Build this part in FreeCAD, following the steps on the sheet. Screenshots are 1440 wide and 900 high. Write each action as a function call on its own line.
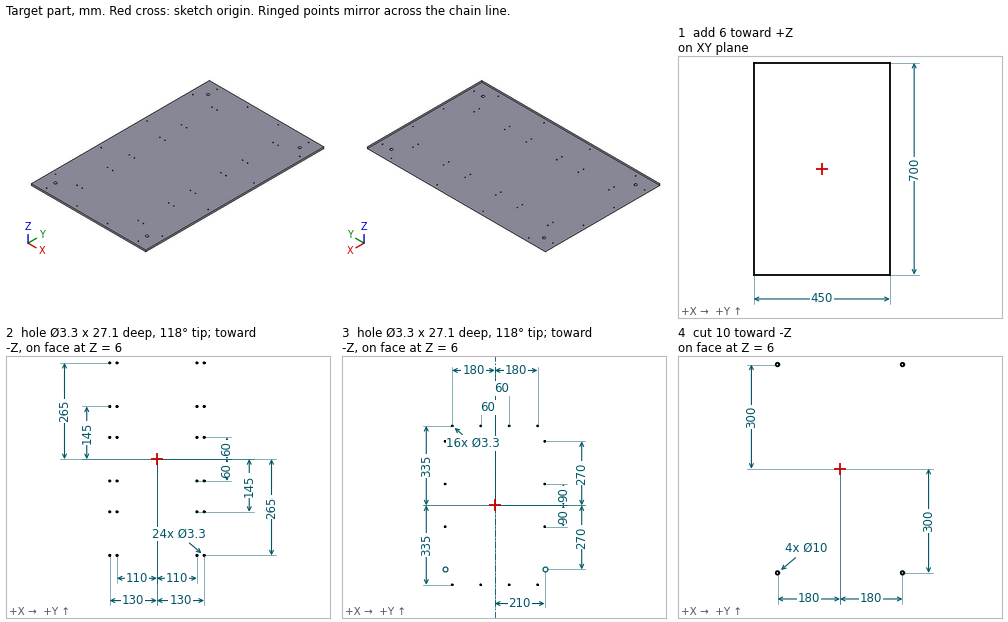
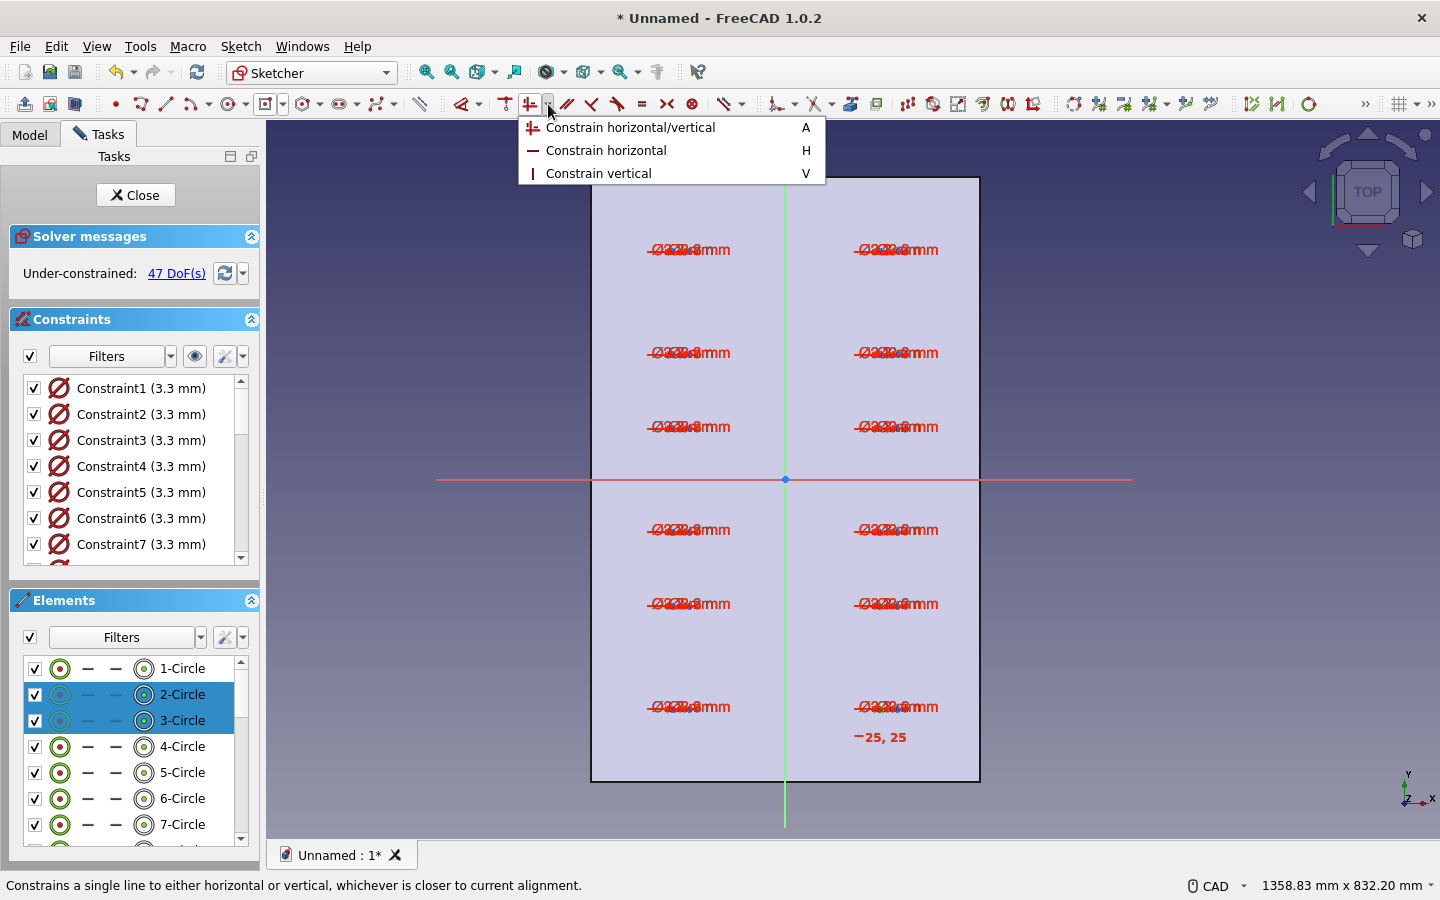
click(672, 174)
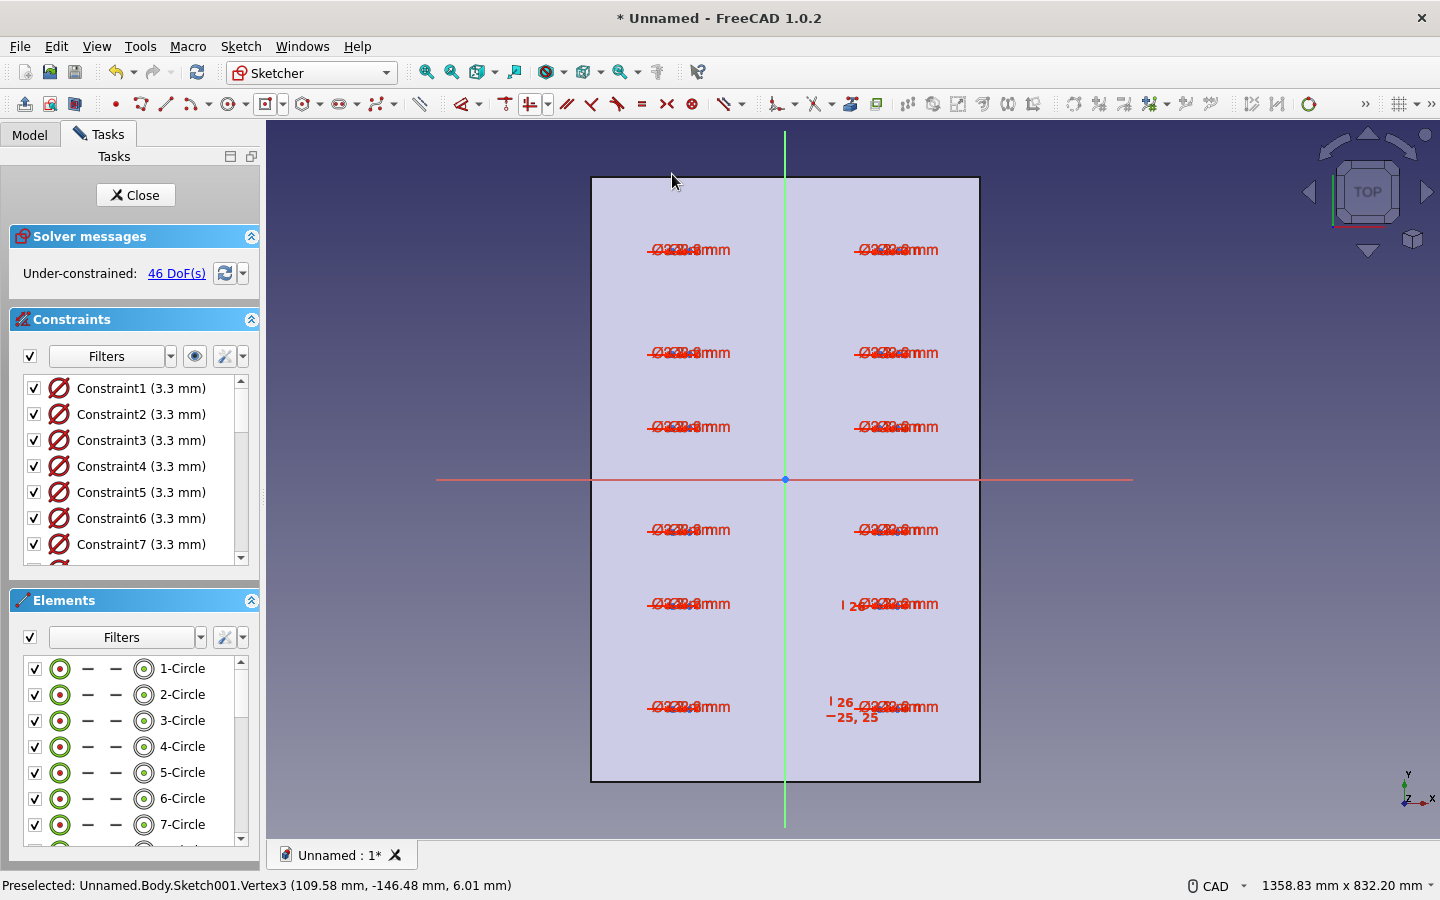
click(898, 709)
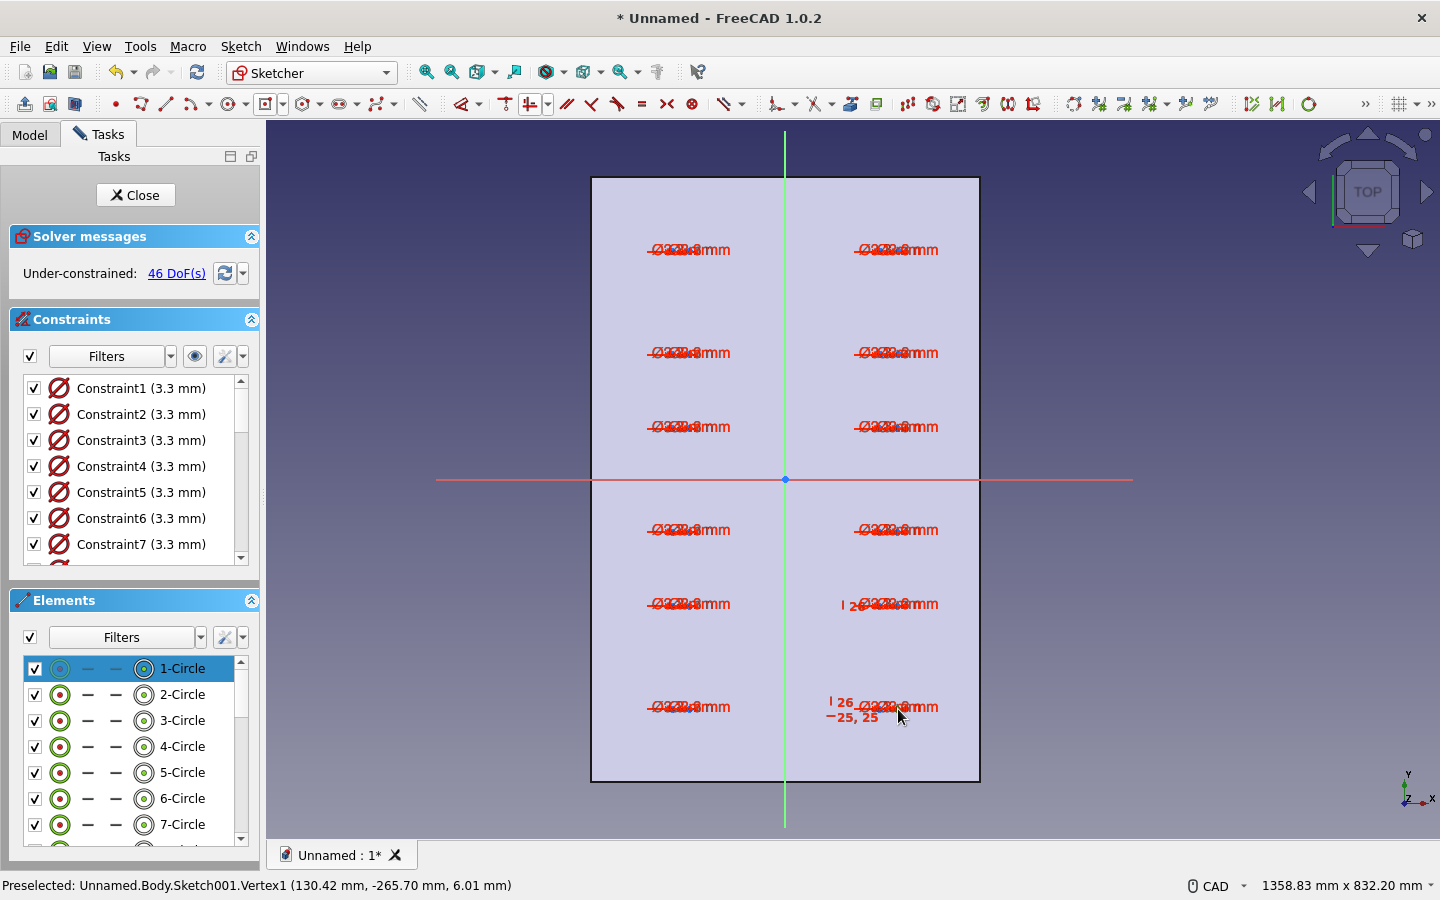
click(898, 606)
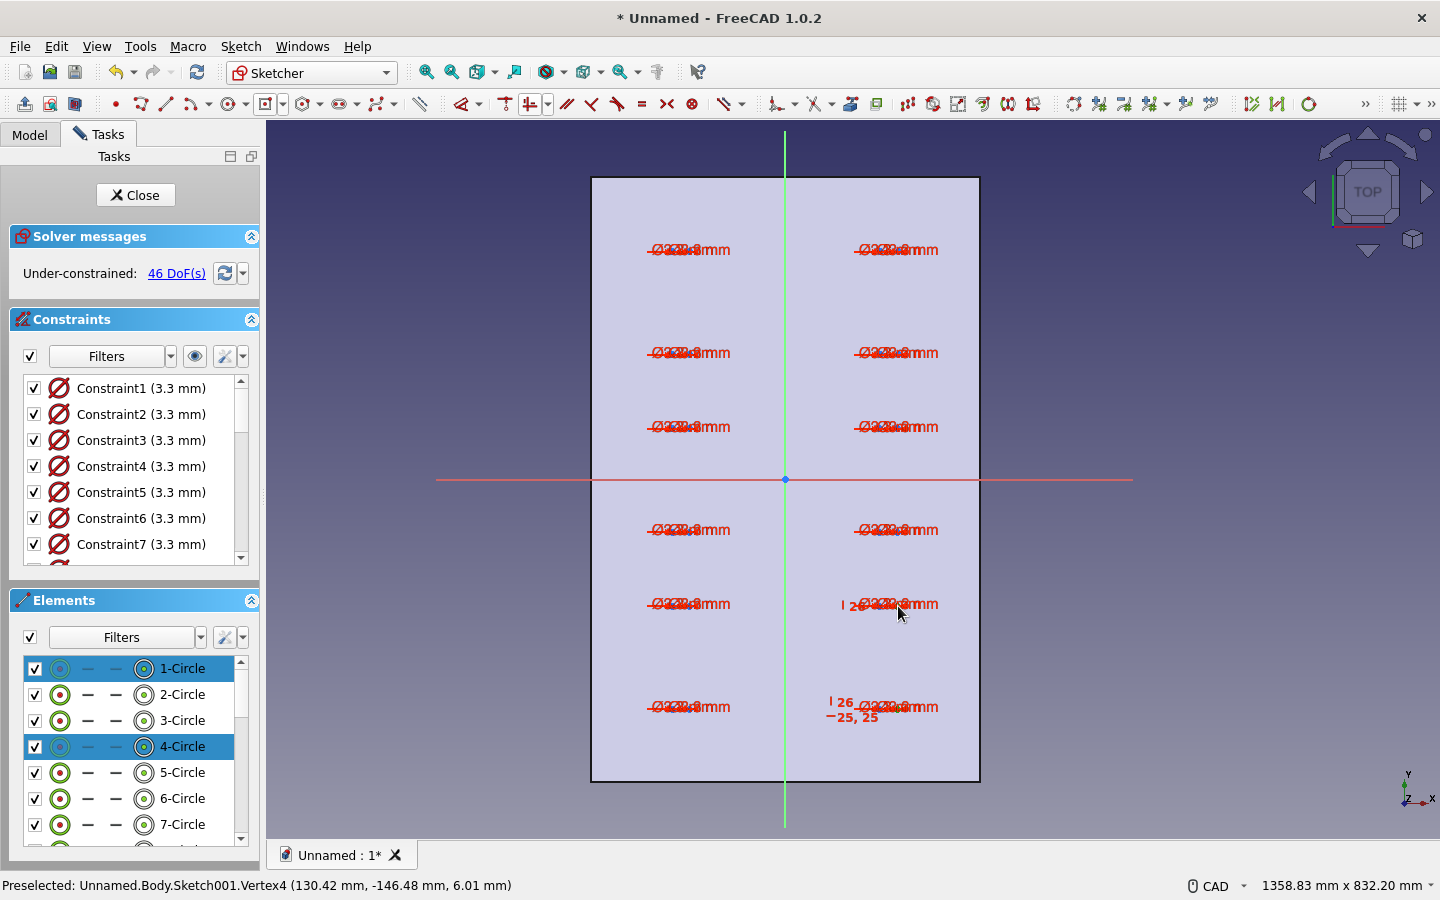
click(548, 104)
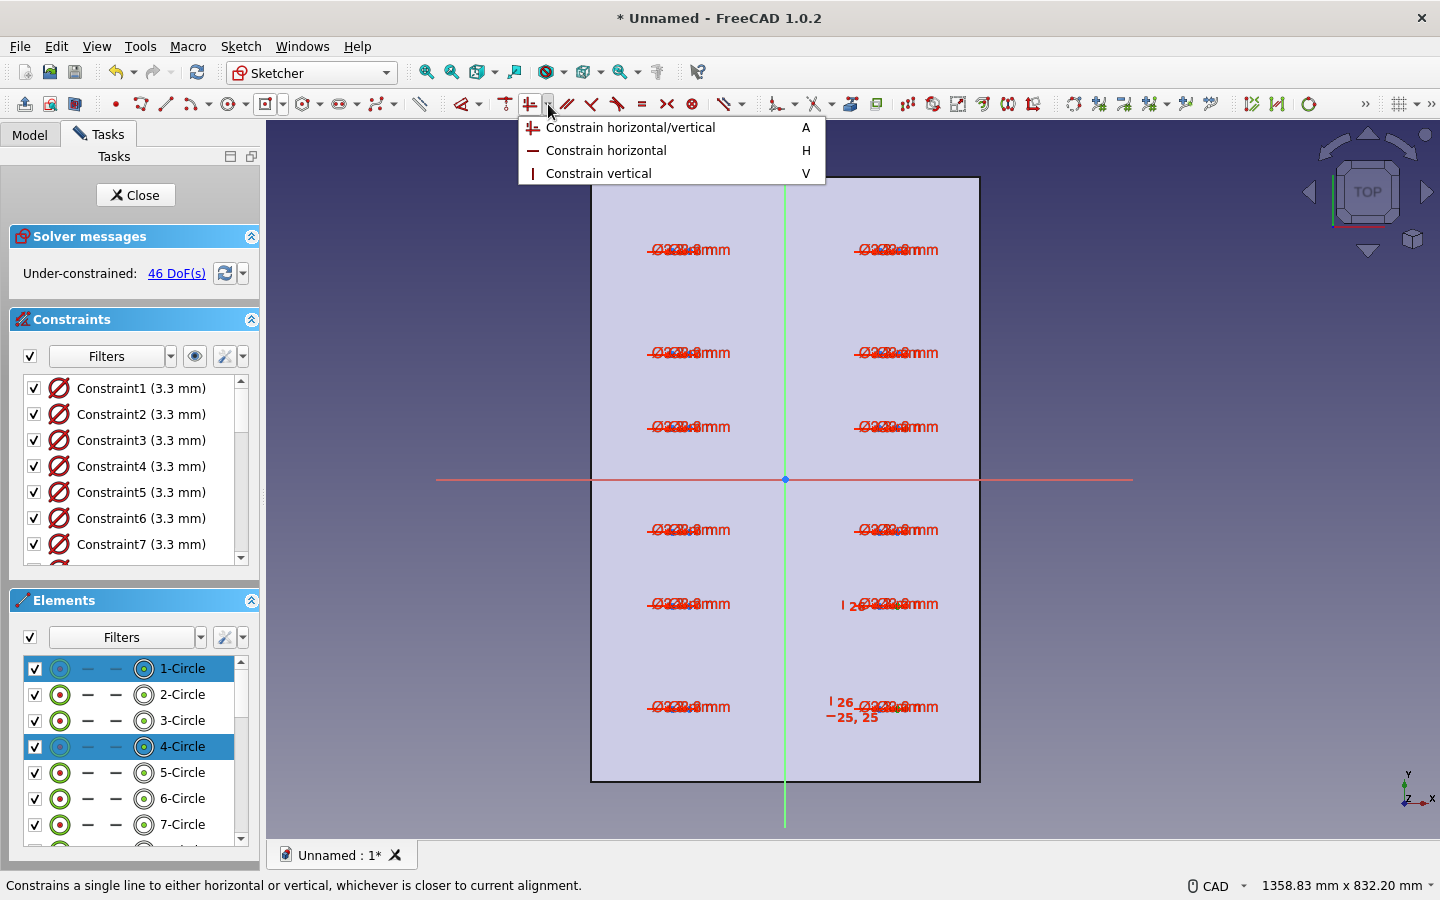
click(672, 174)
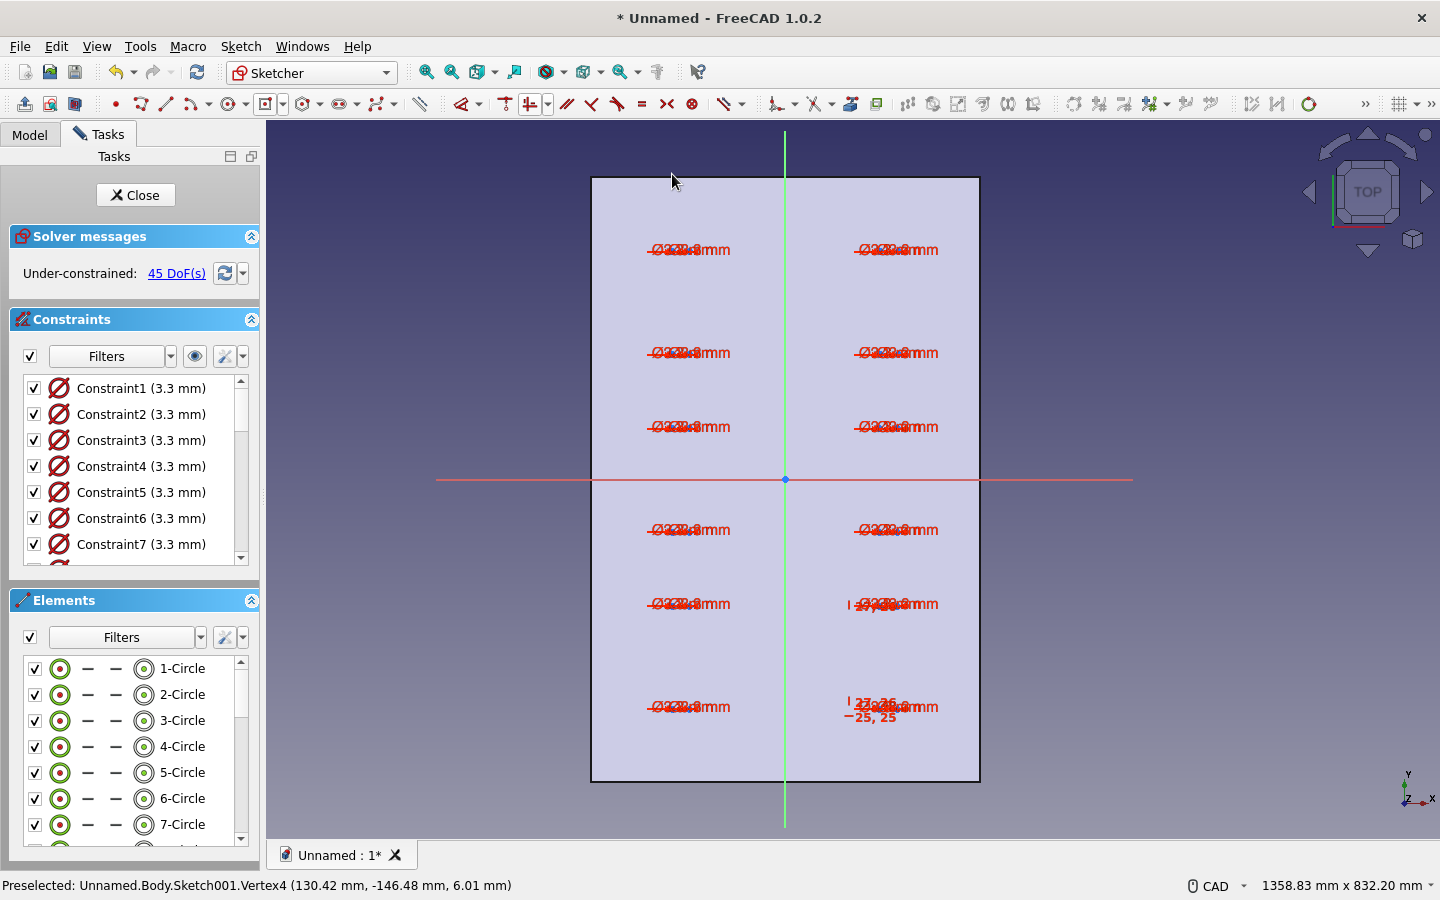
scroll(880, 606, up, 4)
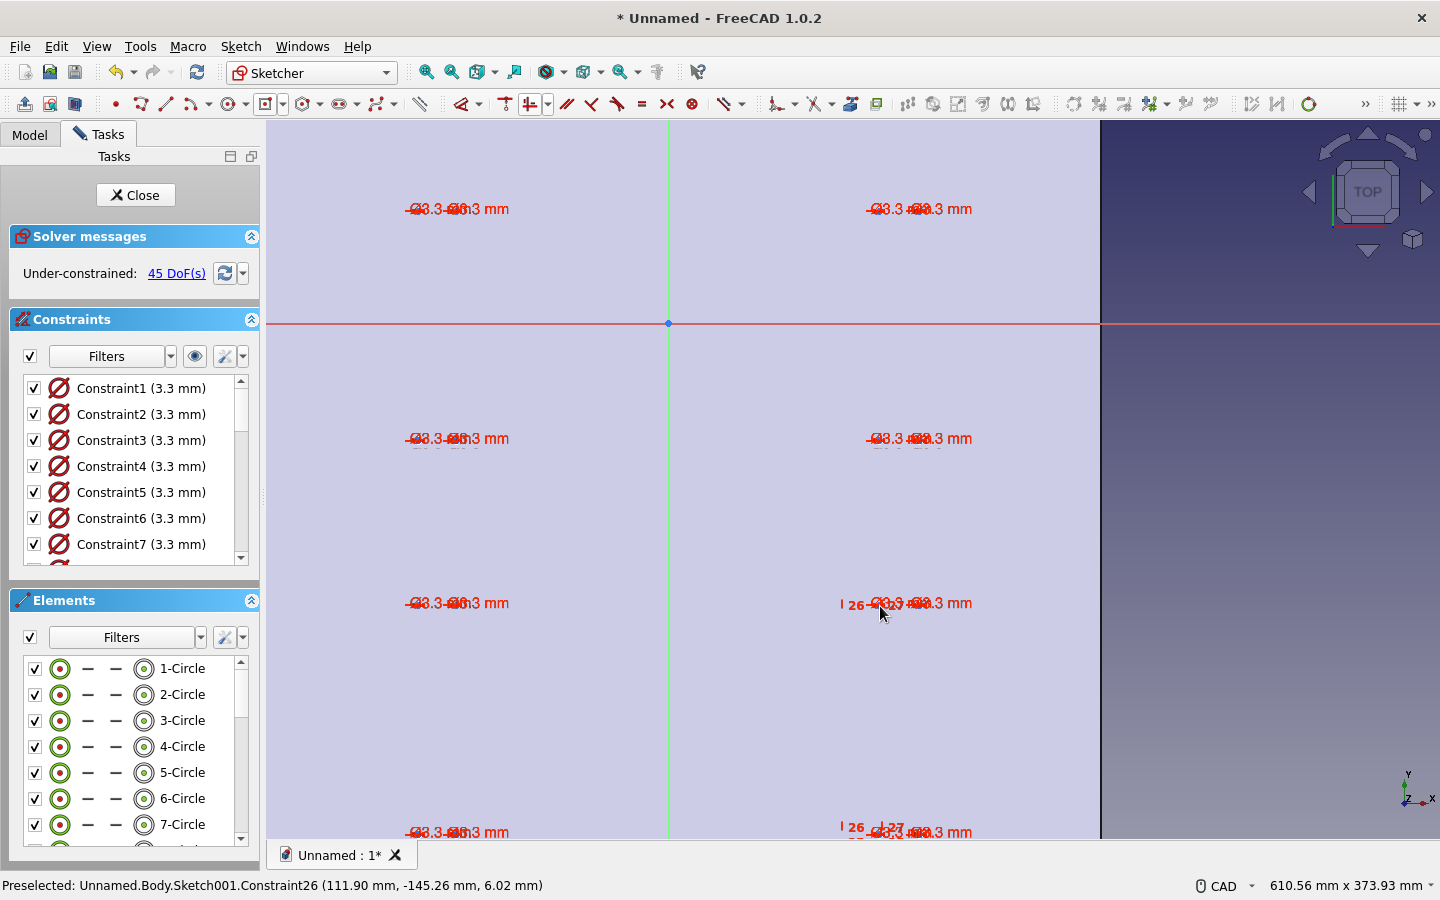
scroll(879, 605, up, 4)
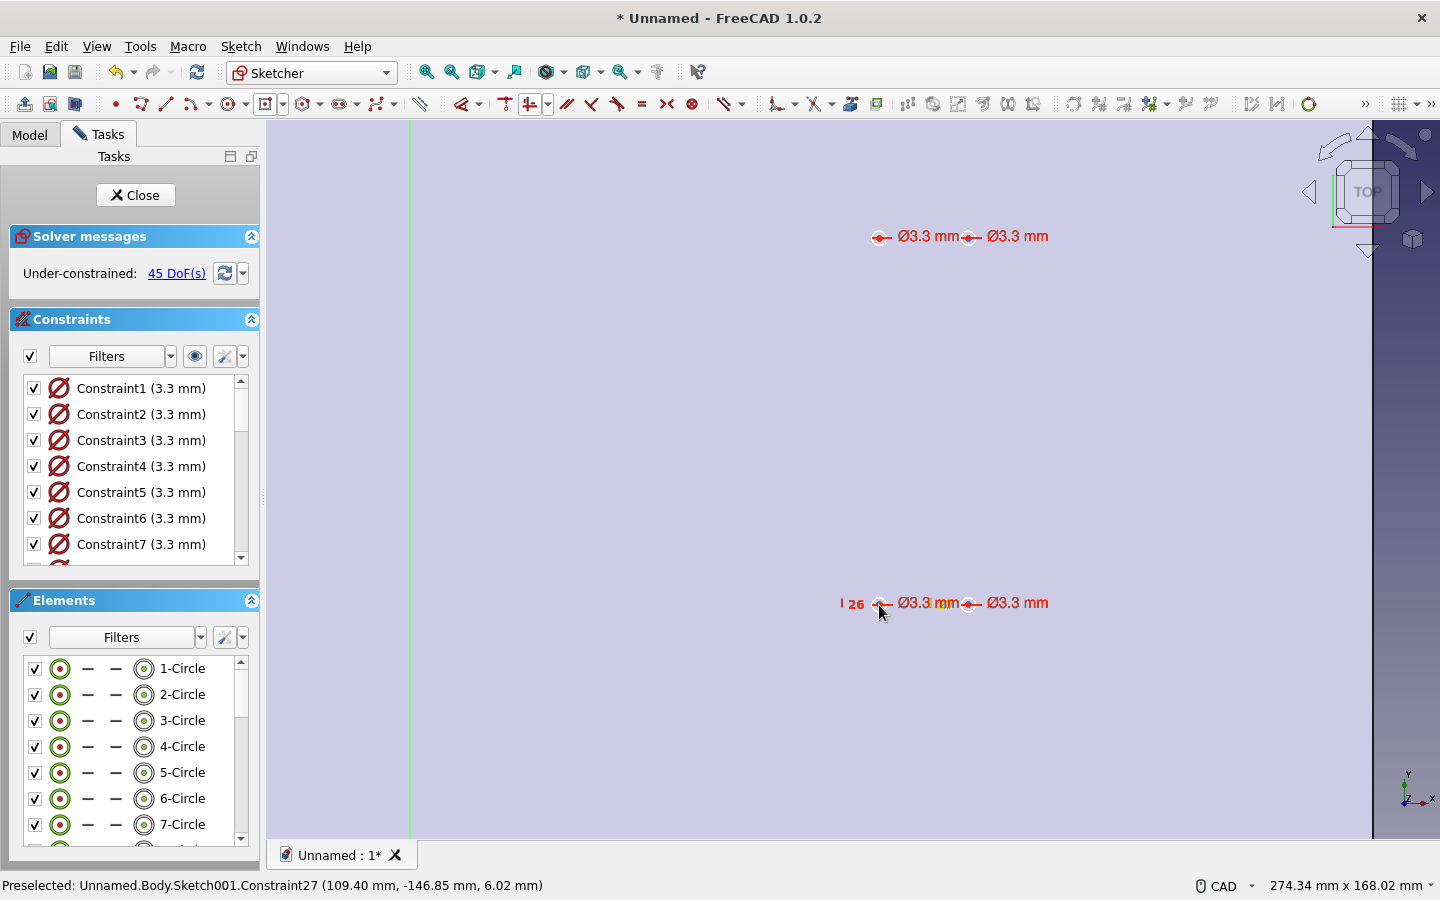
click(879, 605)